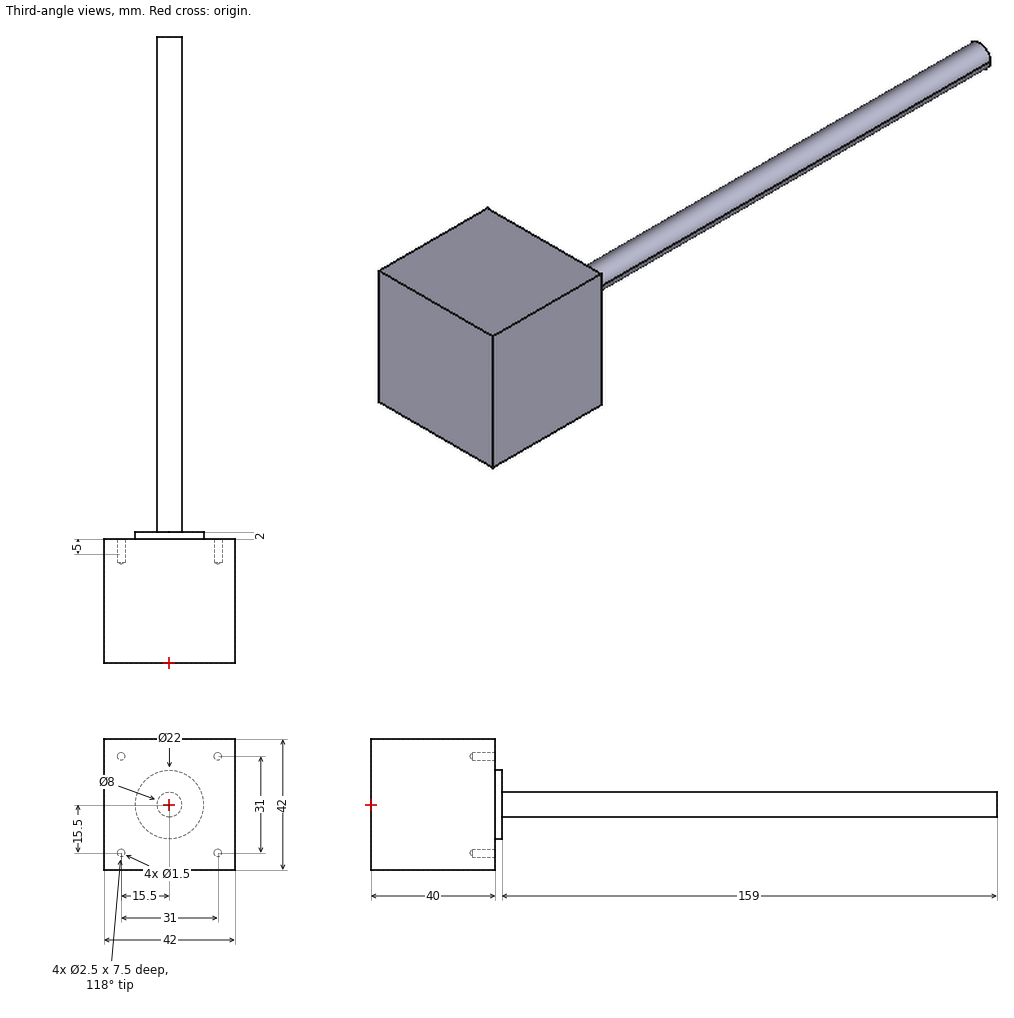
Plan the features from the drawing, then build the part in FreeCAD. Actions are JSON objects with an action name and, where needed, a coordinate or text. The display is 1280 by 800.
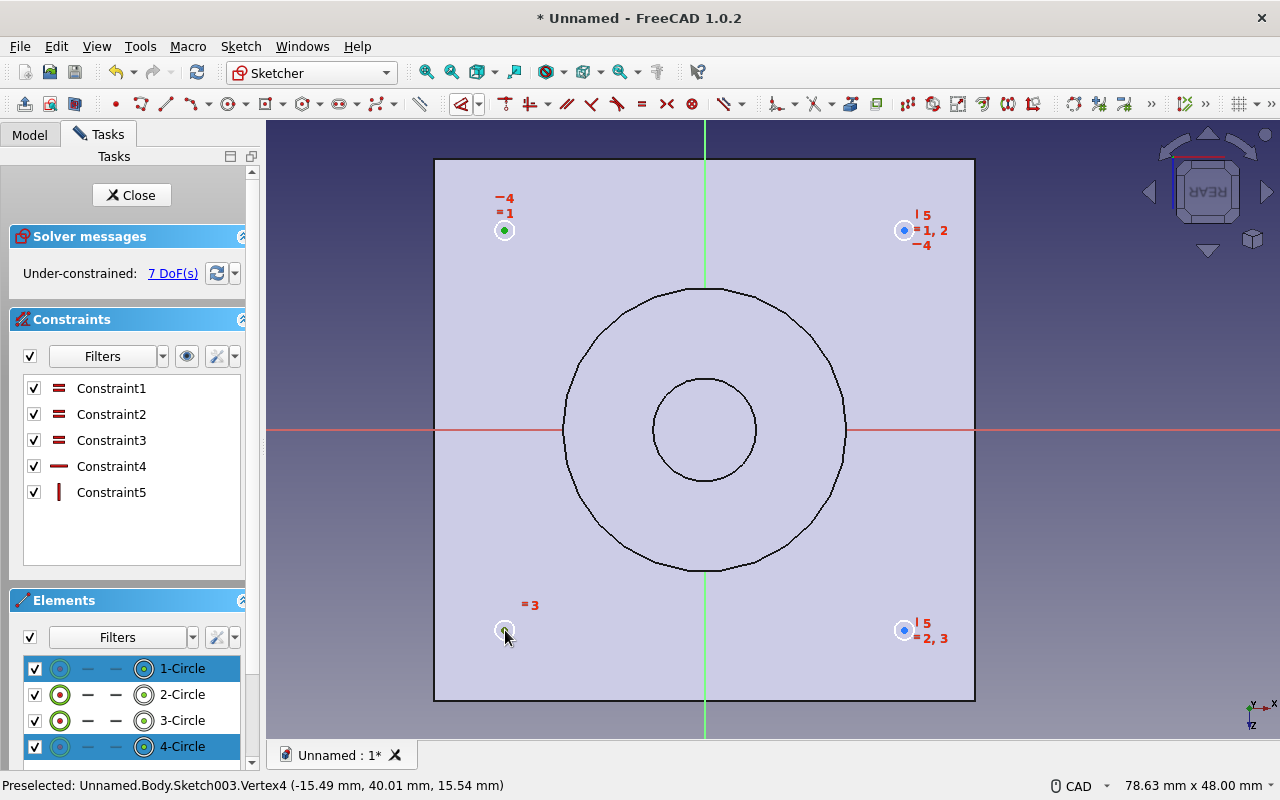
{"action": "left_click", "coordinate": [548, 104]}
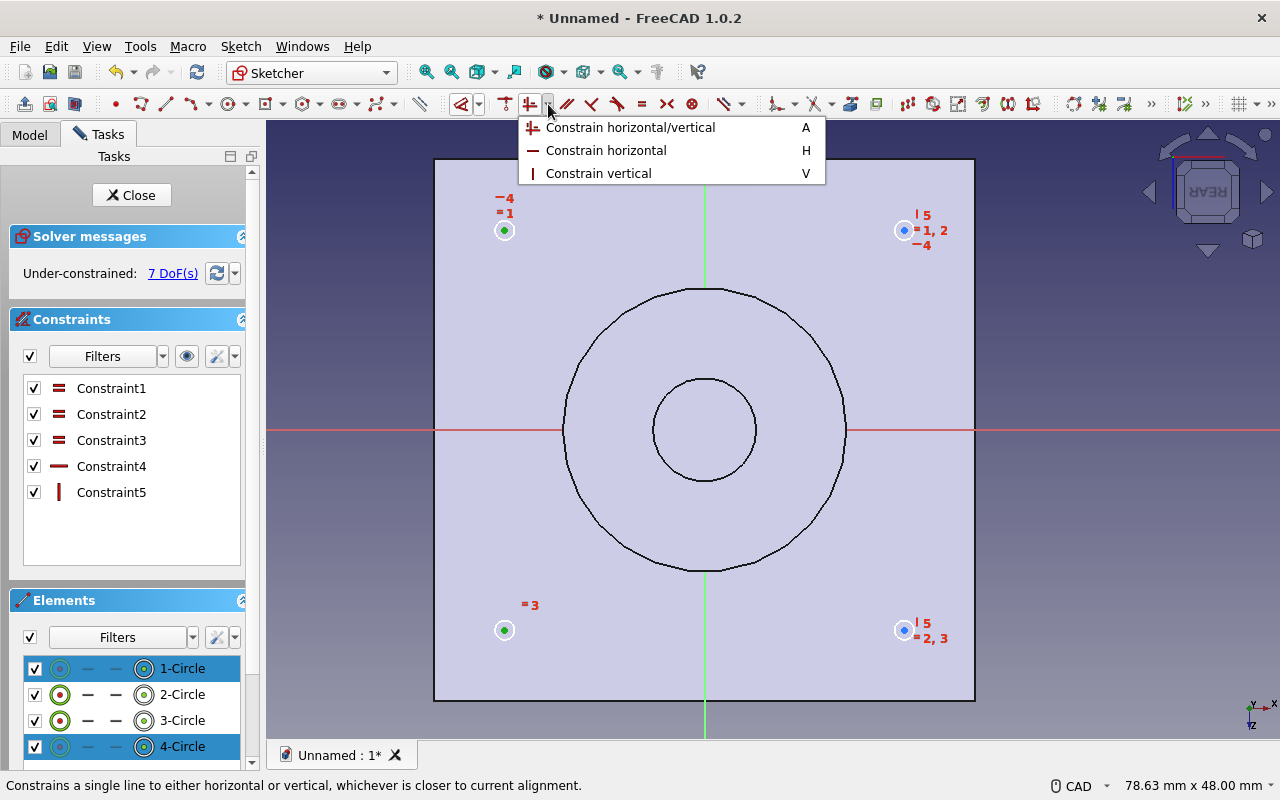
{"action": "left_click", "coordinate": [672, 174]}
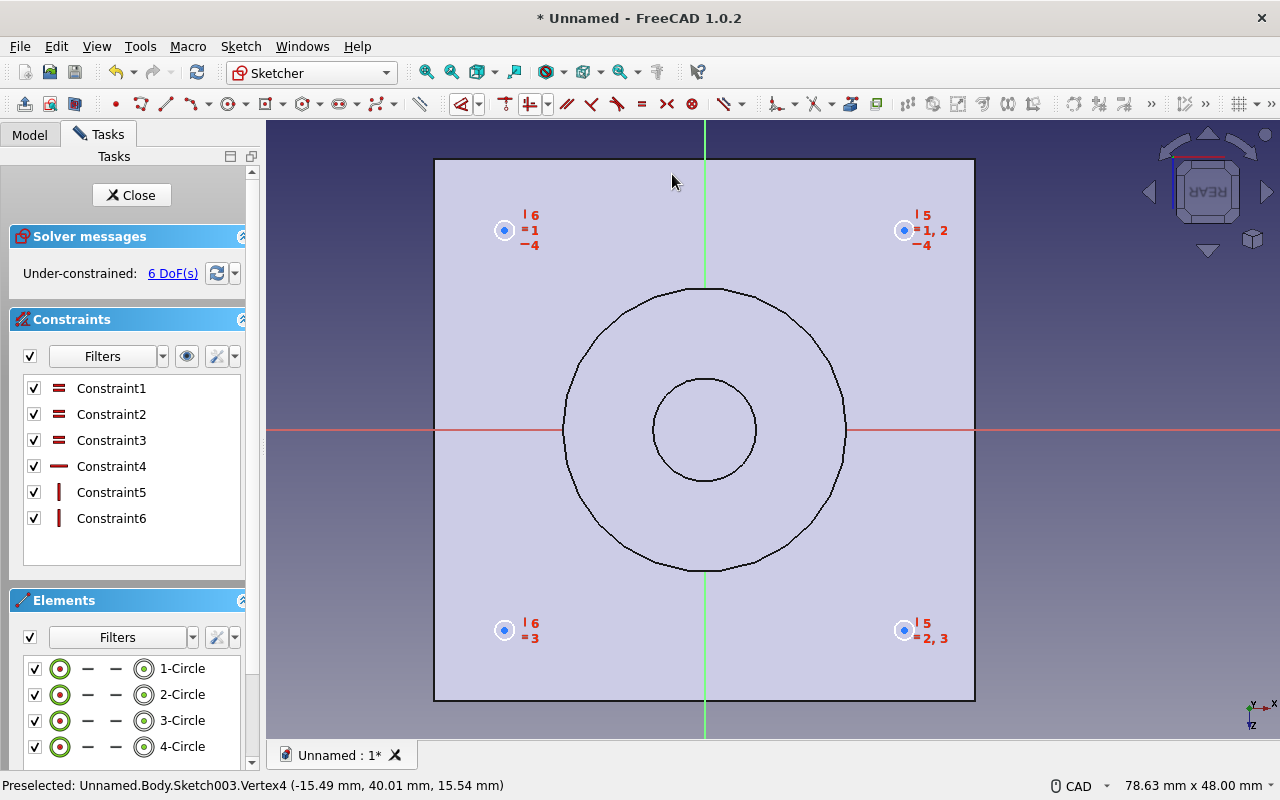
{"action": "left_click", "coordinate": [904, 630]}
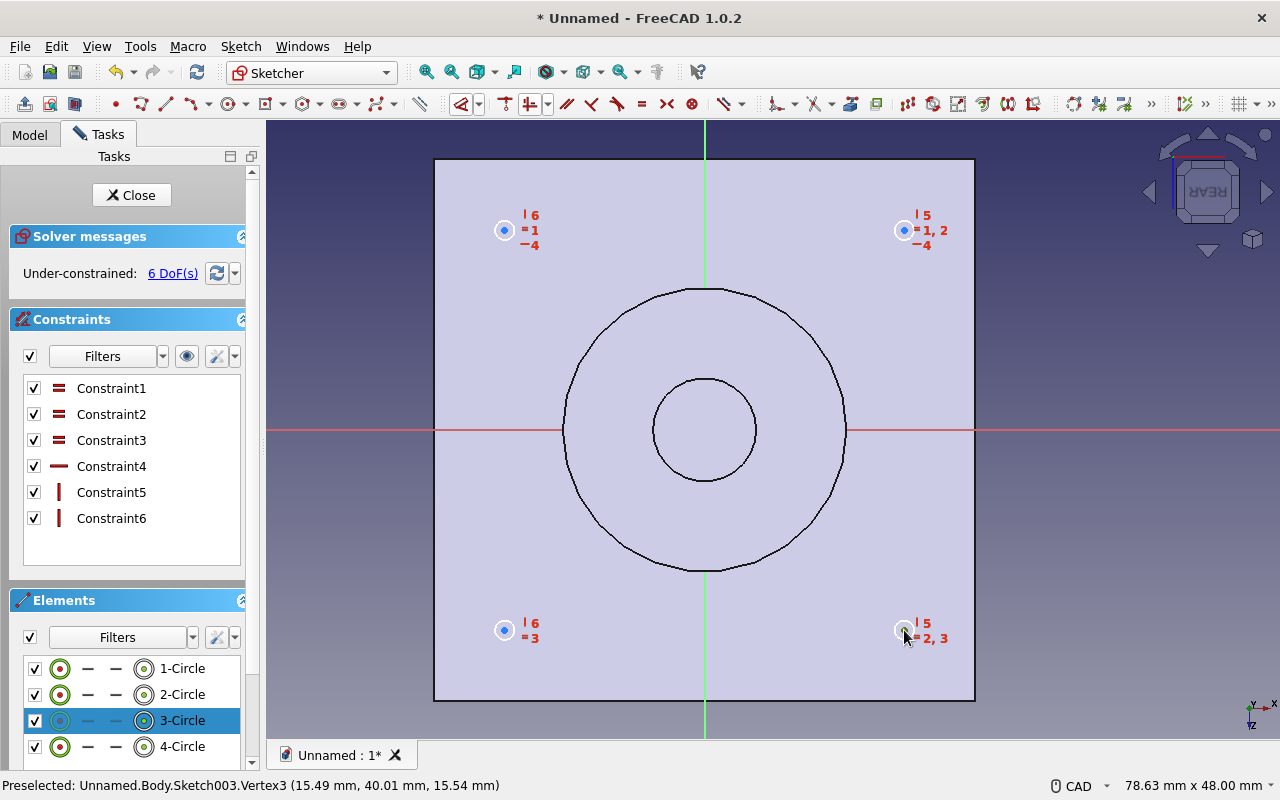
{"action": "left_click", "coordinate": [505, 630]}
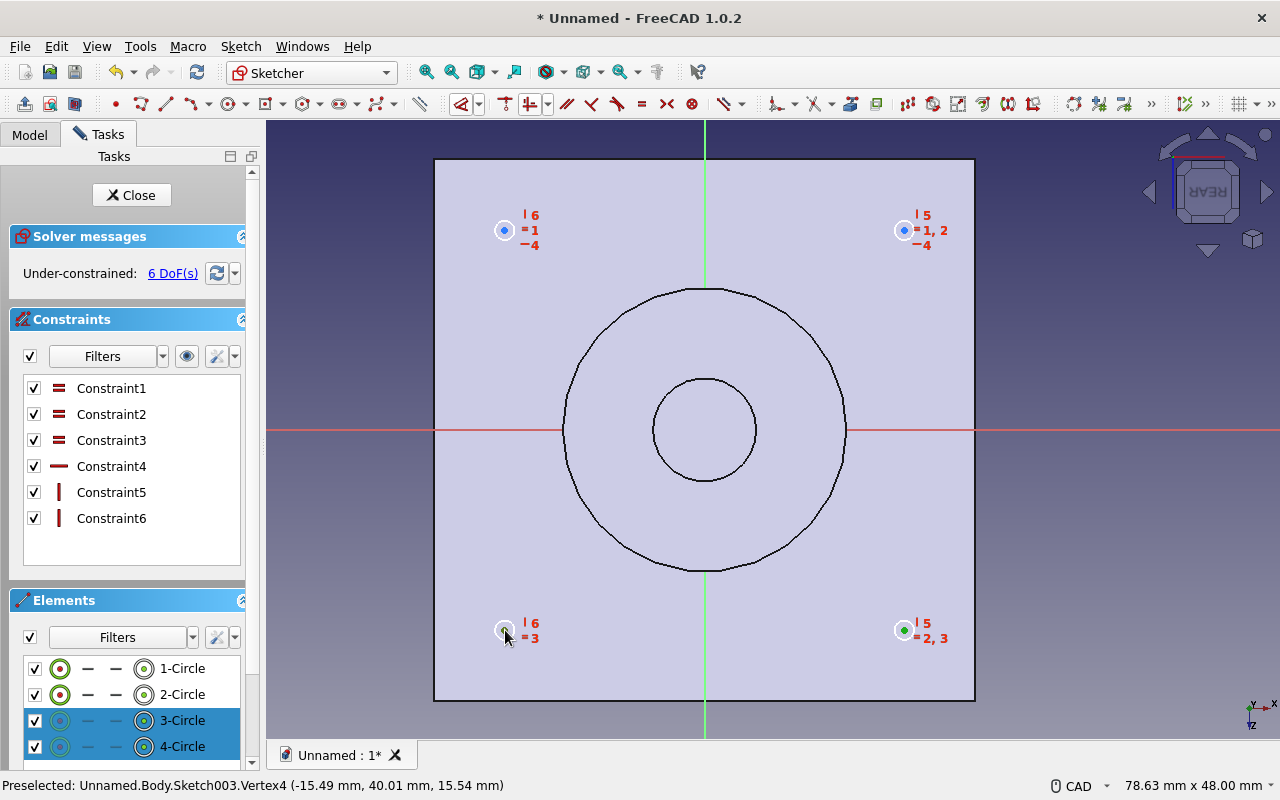
{"action": "key", "text": "h"}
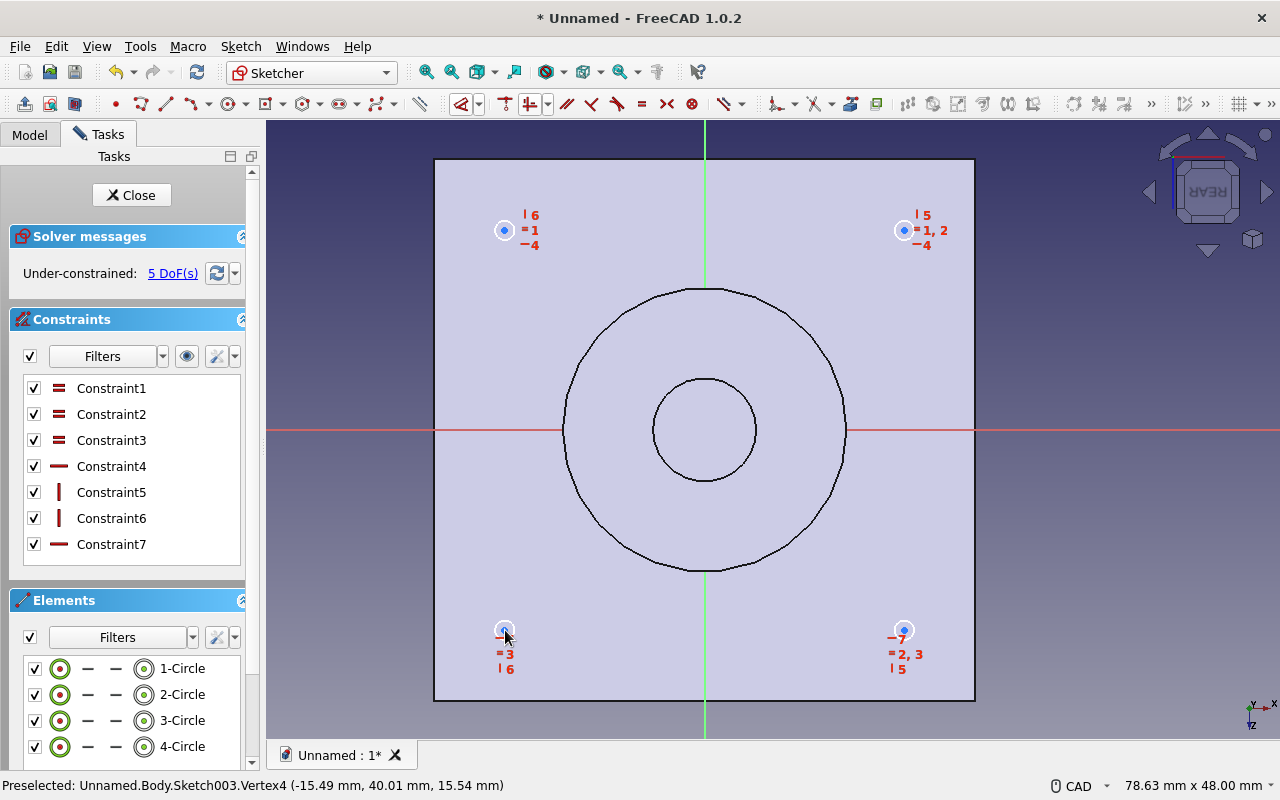
{"action": "scroll", "coordinate": [512, 224], "scroll_direction": "up", "scroll_amount": 4}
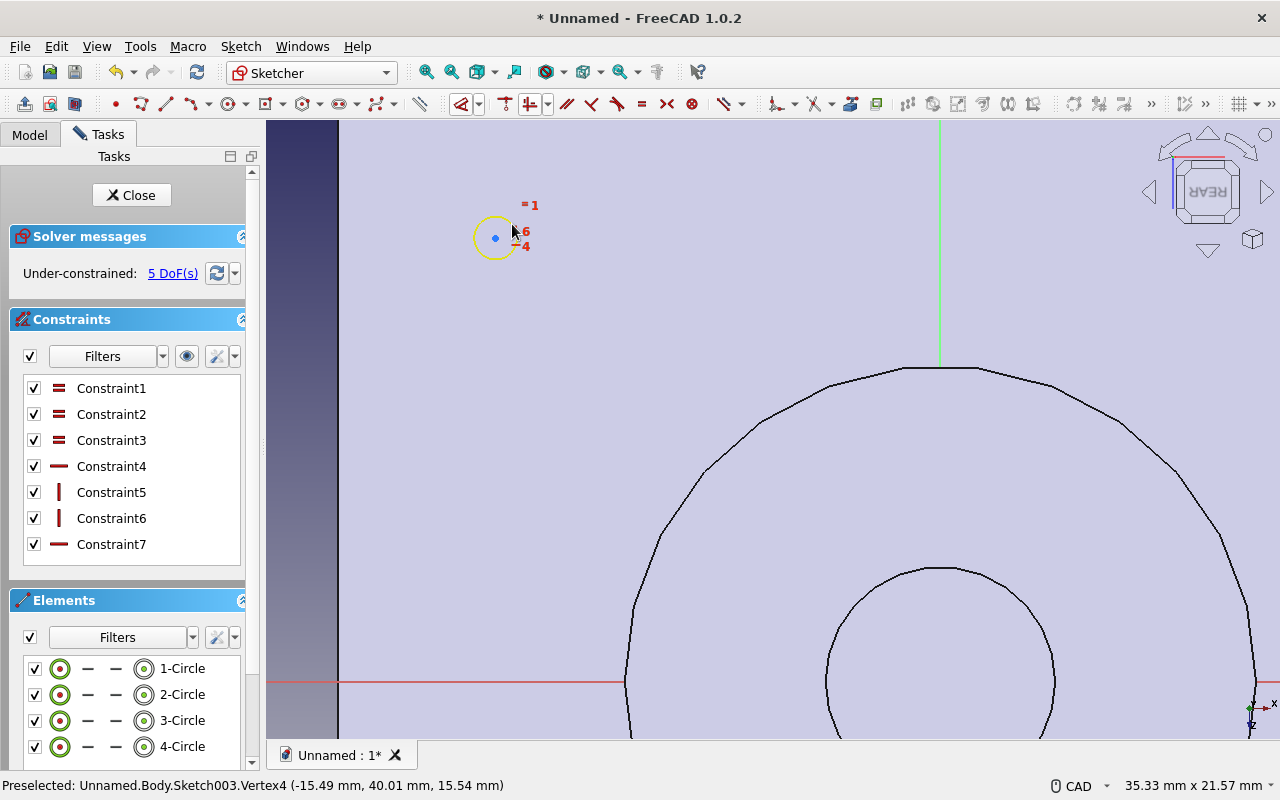
{"action": "left_click", "coordinate": [481, 223]}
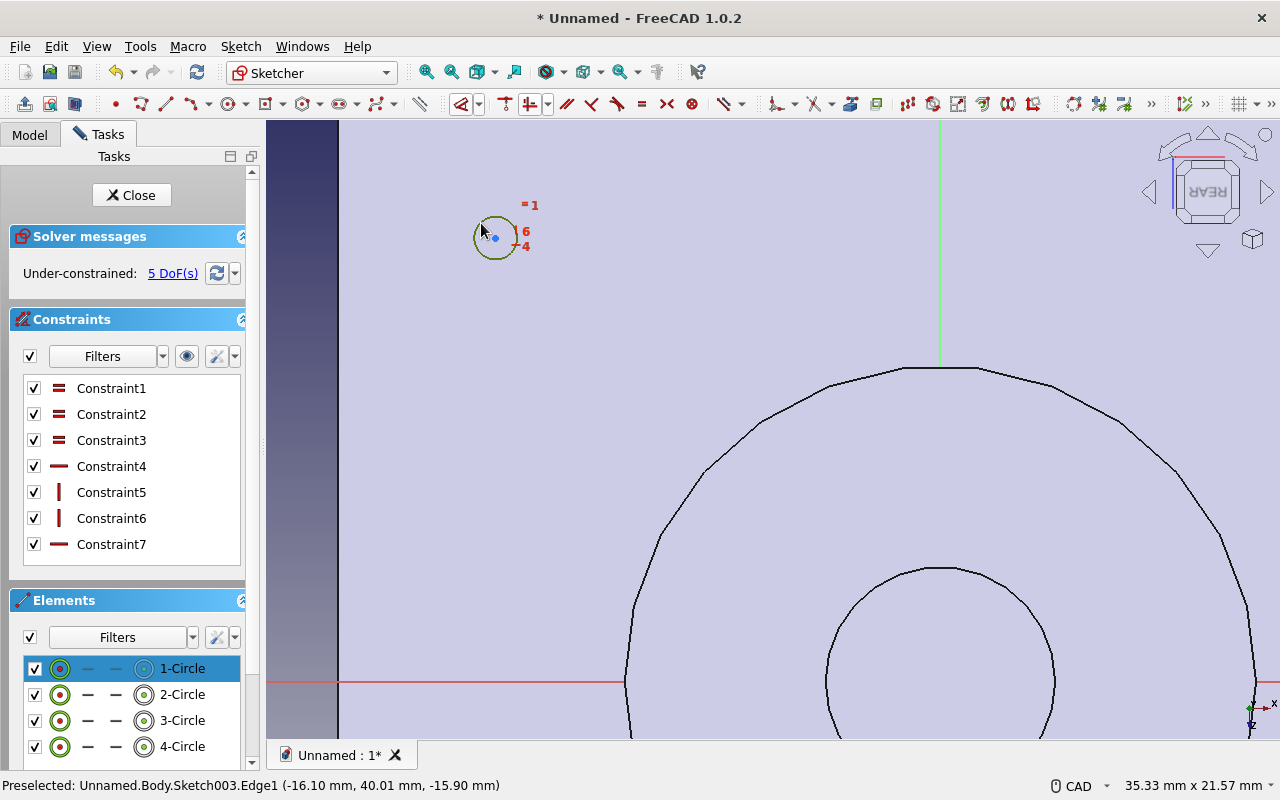
{"action": "key", "text": "k o"}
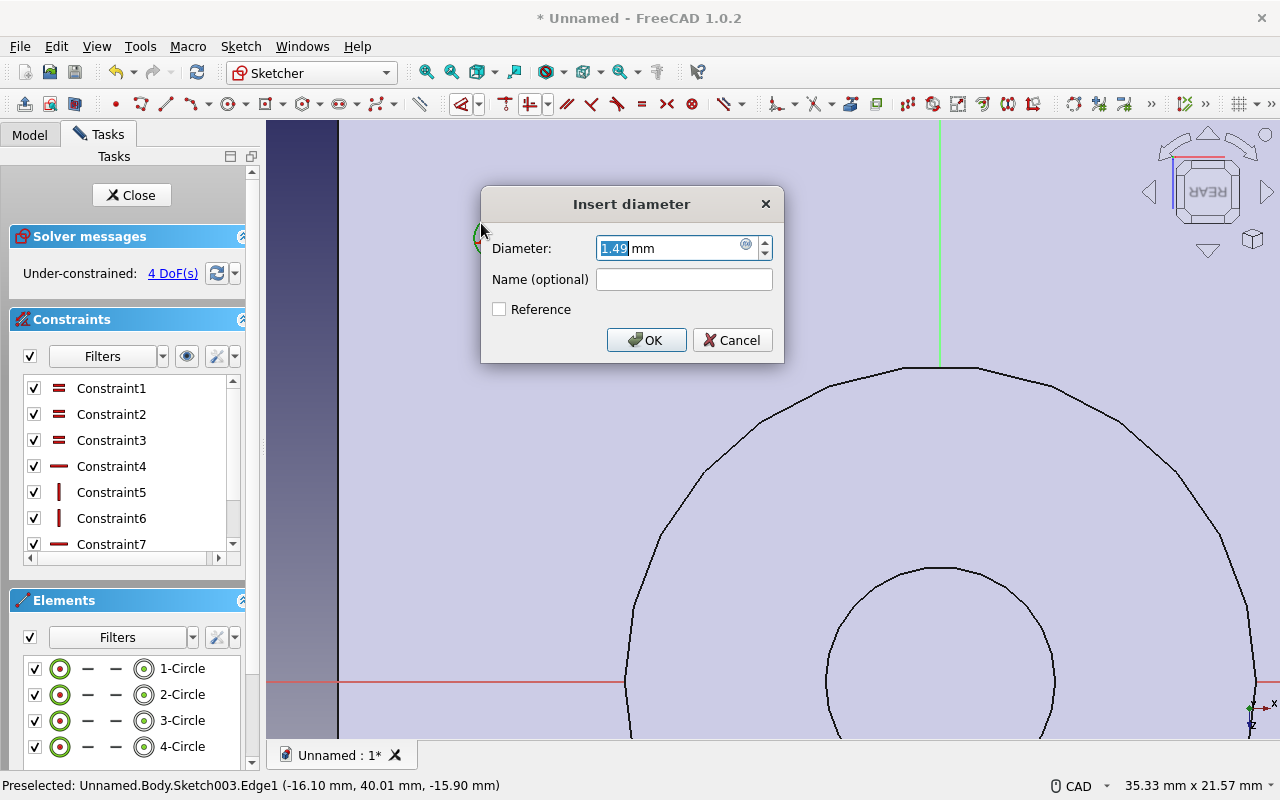
{"action": "type", "text": "1.5"}
{"action": "key", "text": "Return"}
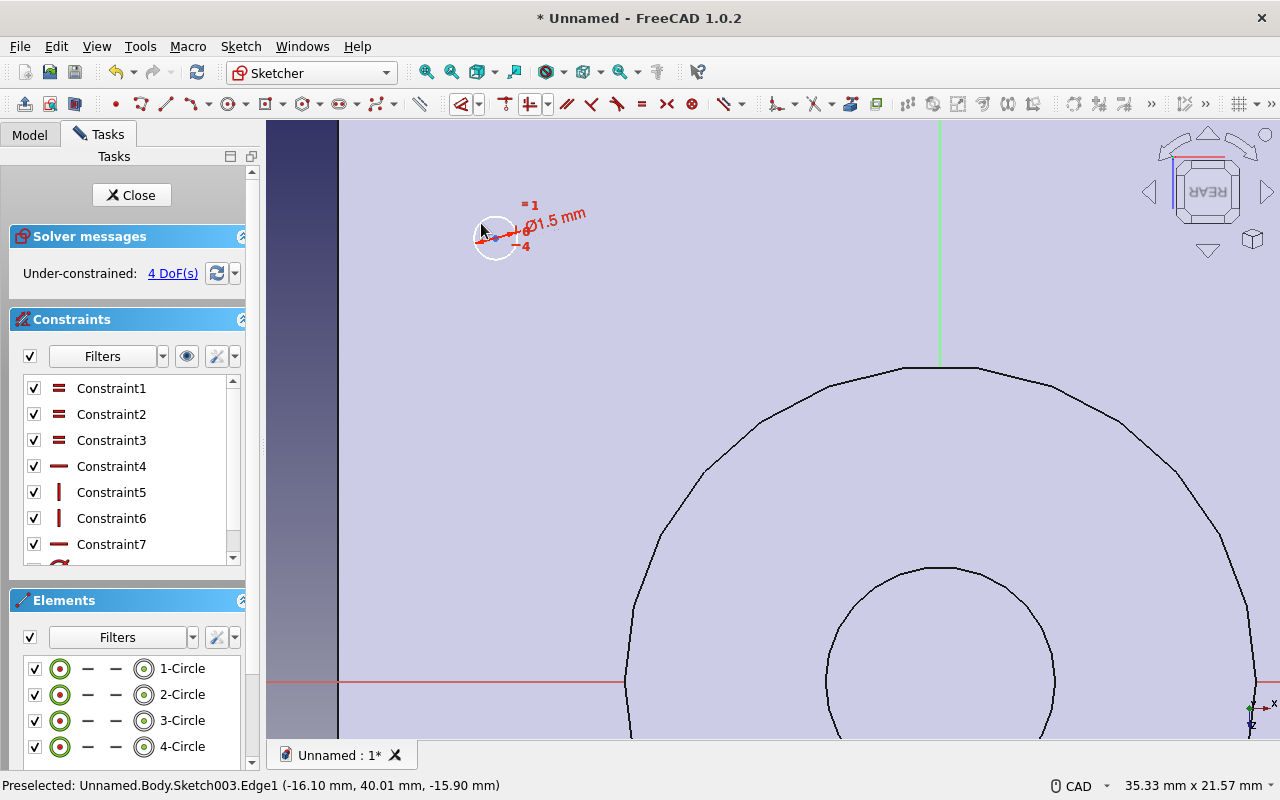
{"action": "left_click", "coordinate": [496, 238]}